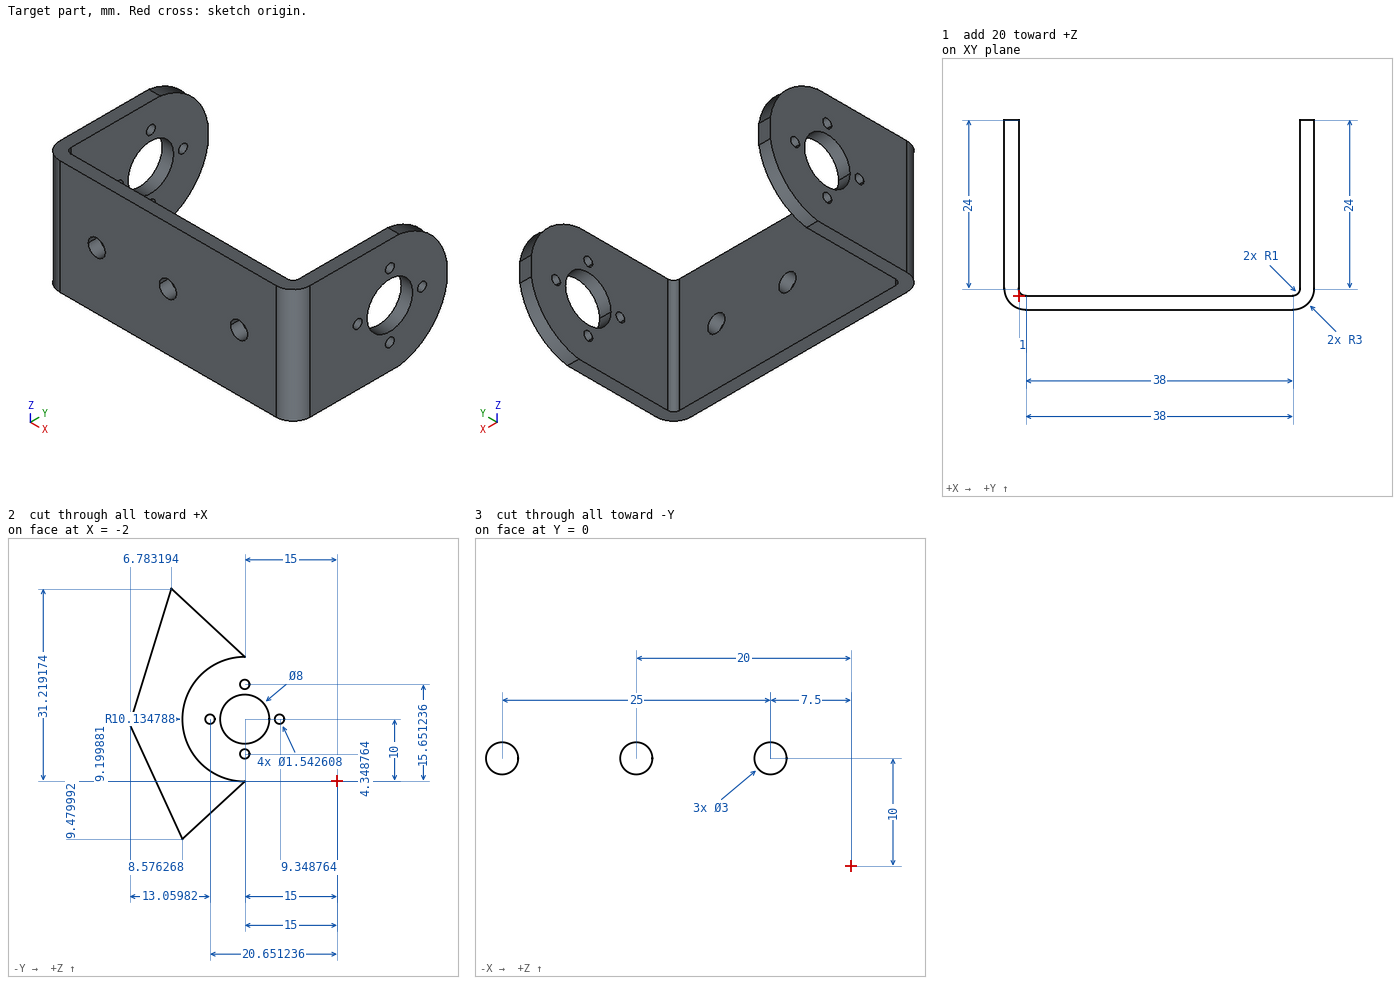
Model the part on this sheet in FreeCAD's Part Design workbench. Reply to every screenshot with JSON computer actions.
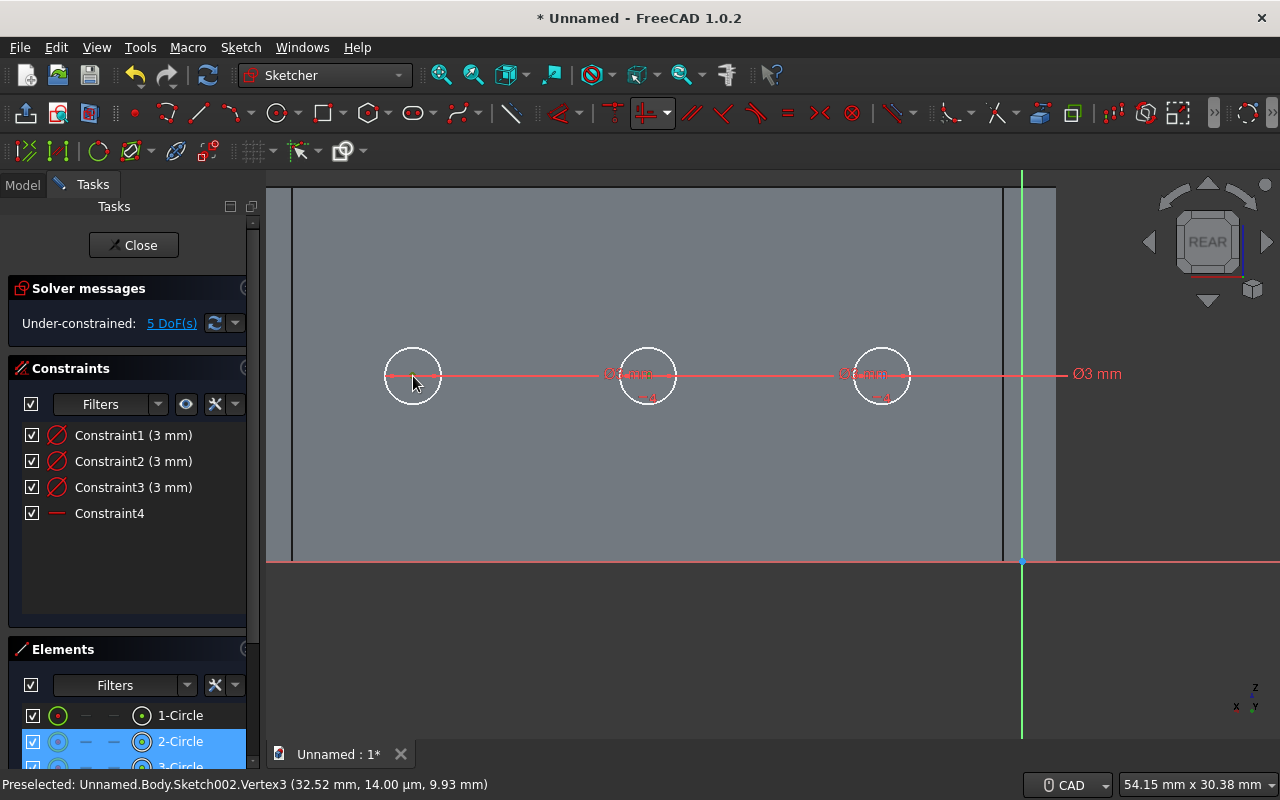
{"action": "left_click", "coordinate": [670, 114]}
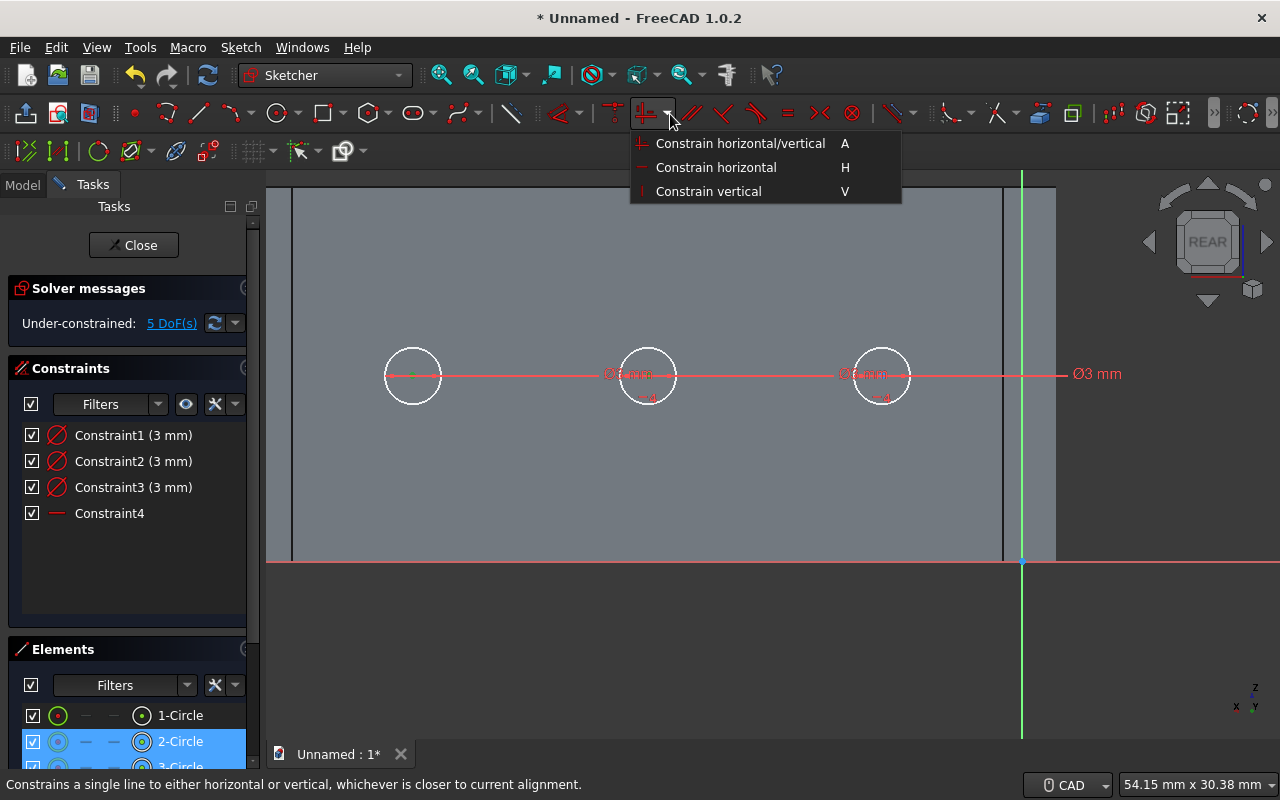
{"action": "left_click", "coordinate": [766, 167]}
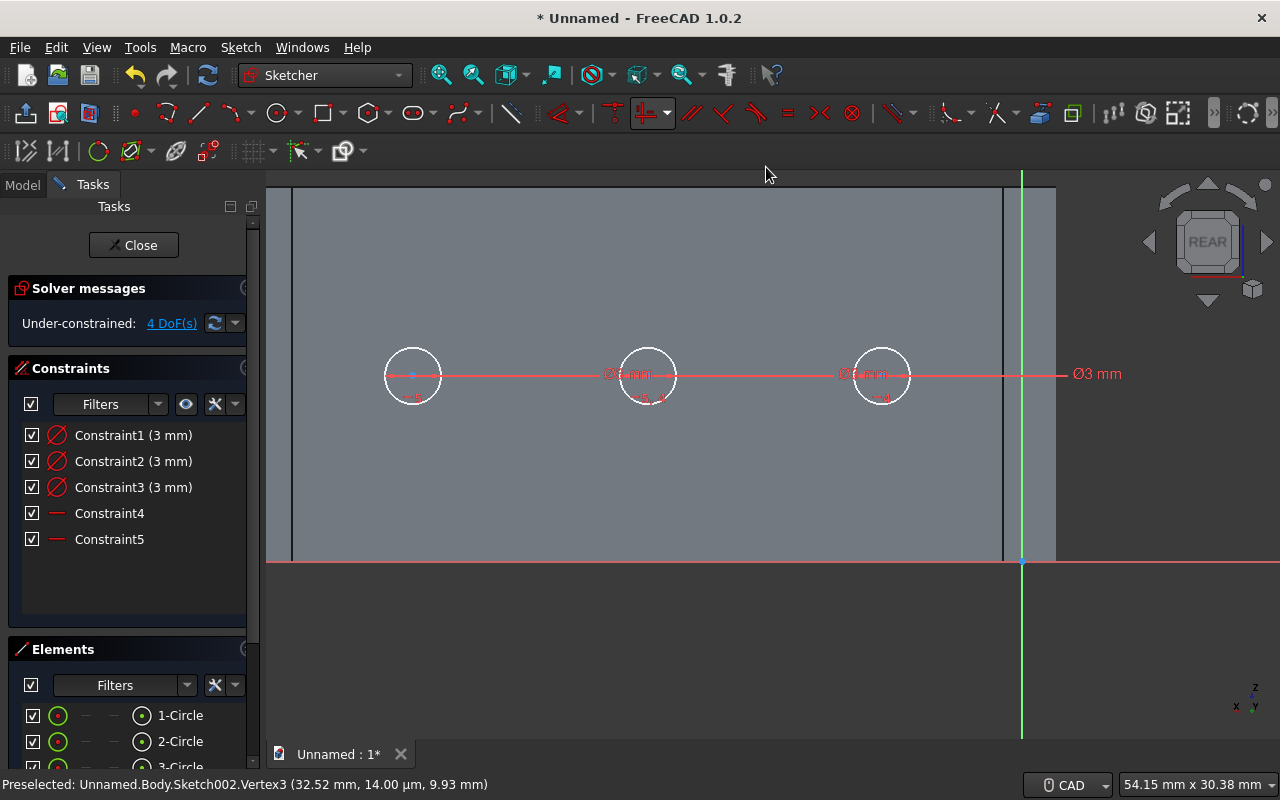
{"action": "left_click", "coordinate": [558, 114]}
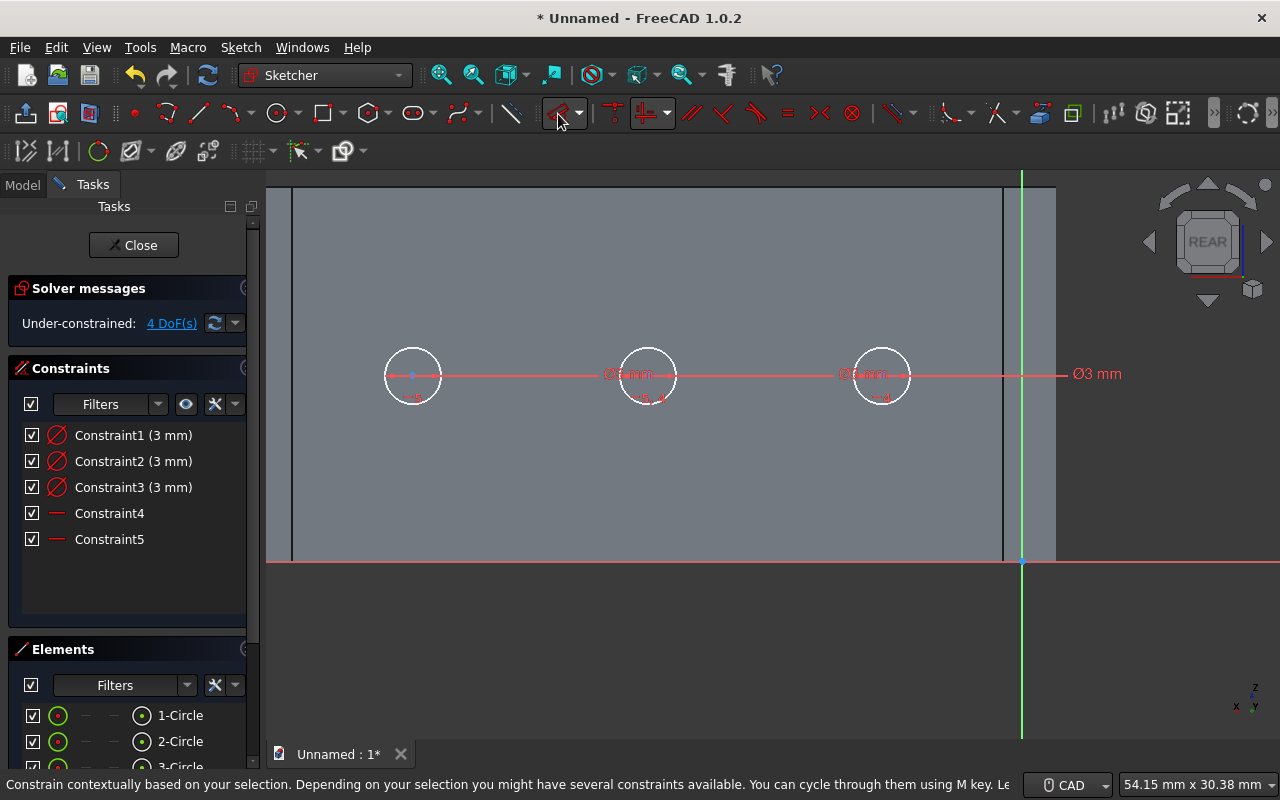
{"action": "left_click", "coordinate": [882, 376]}
{"action": "left_click", "coordinate": [1056, 469]}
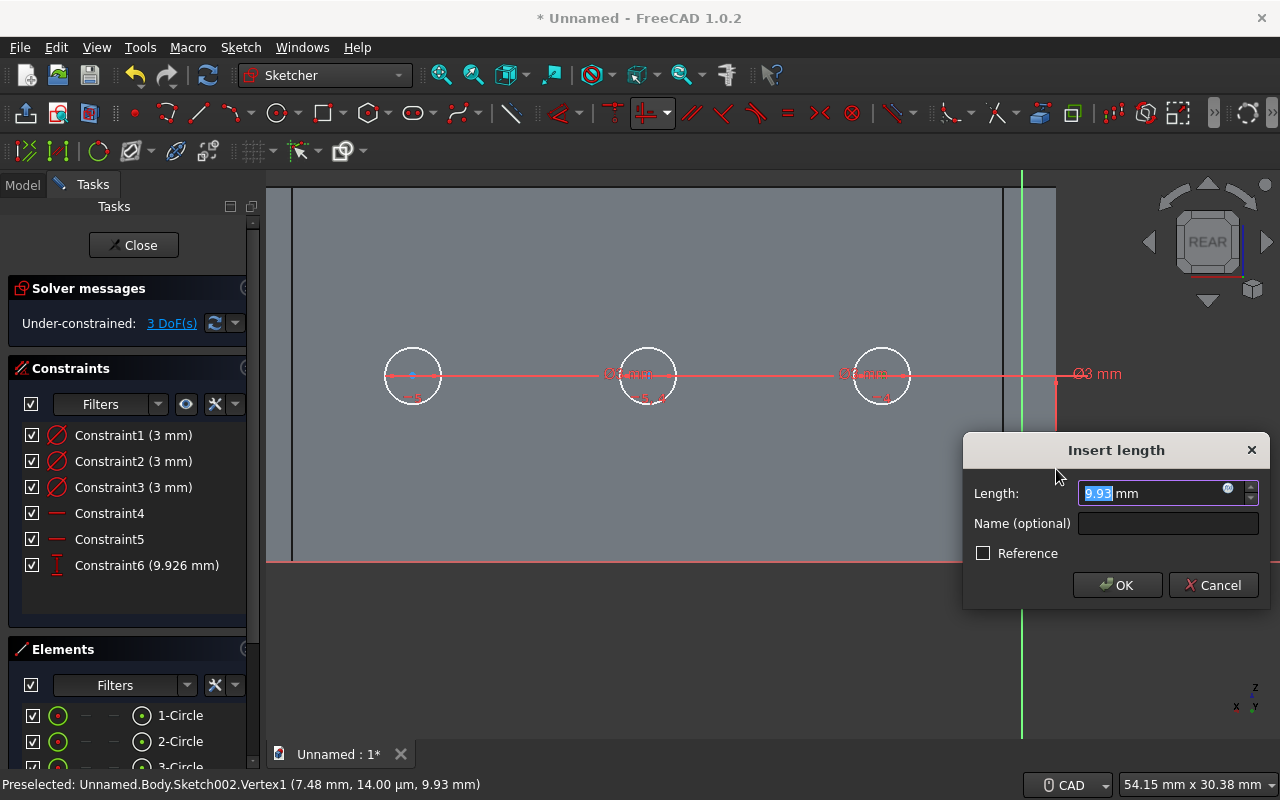
{"action": "type", "text": "10"}
{"action": "key", "text": "Return"}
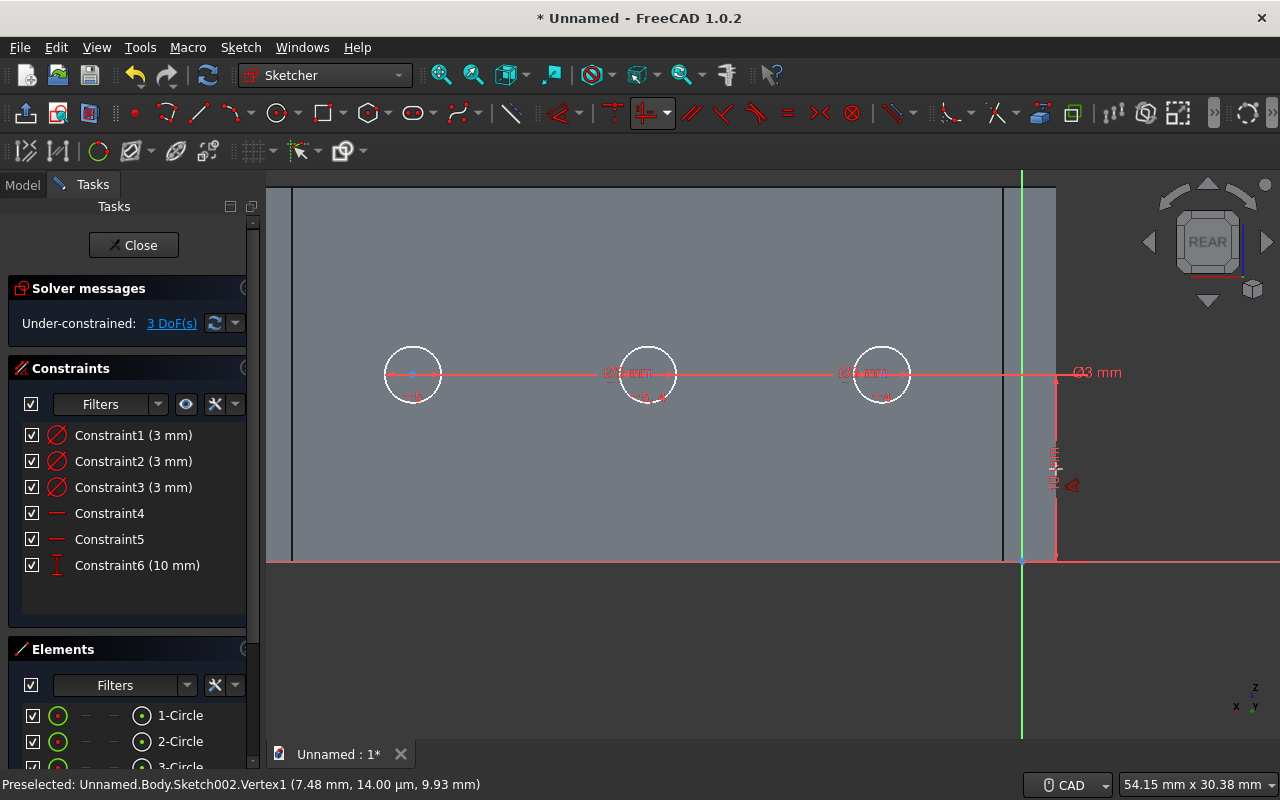
{"action": "left_click", "coordinate": [648, 375]}
{"action": "left_click", "coordinate": [835, 596]}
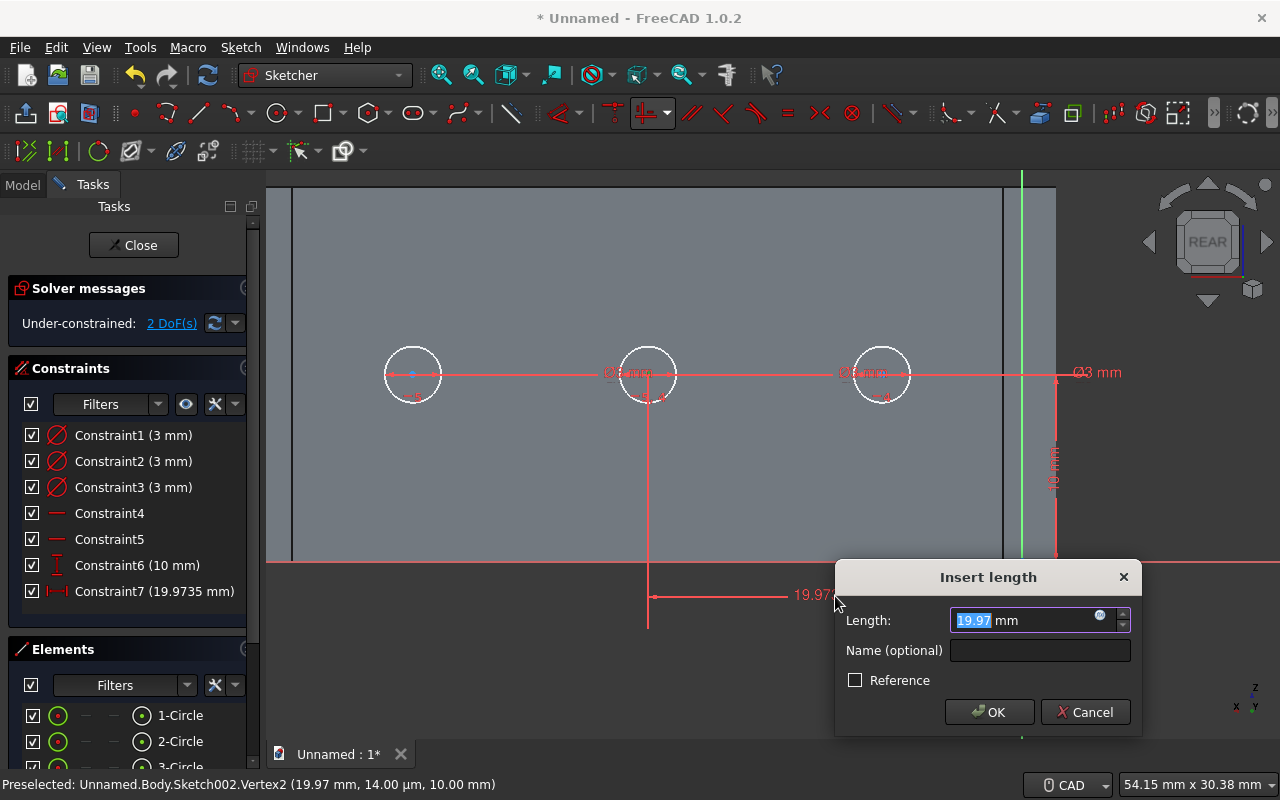
{"action": "type", "text": "20"}
{"action": "key", "text": "Return"}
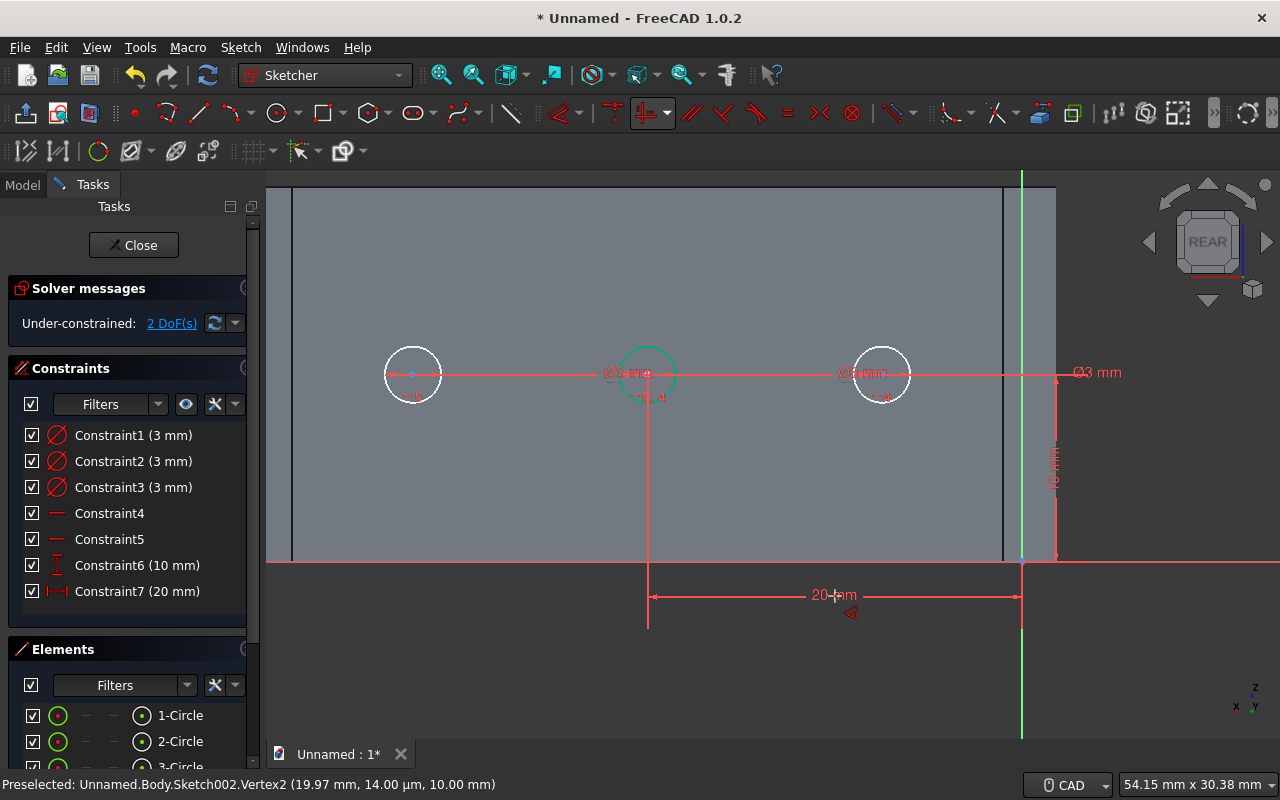
{"action": "left_click", "coordinate": [882, 375]}
{"action": "left_click", "coordinate": [952, 596]}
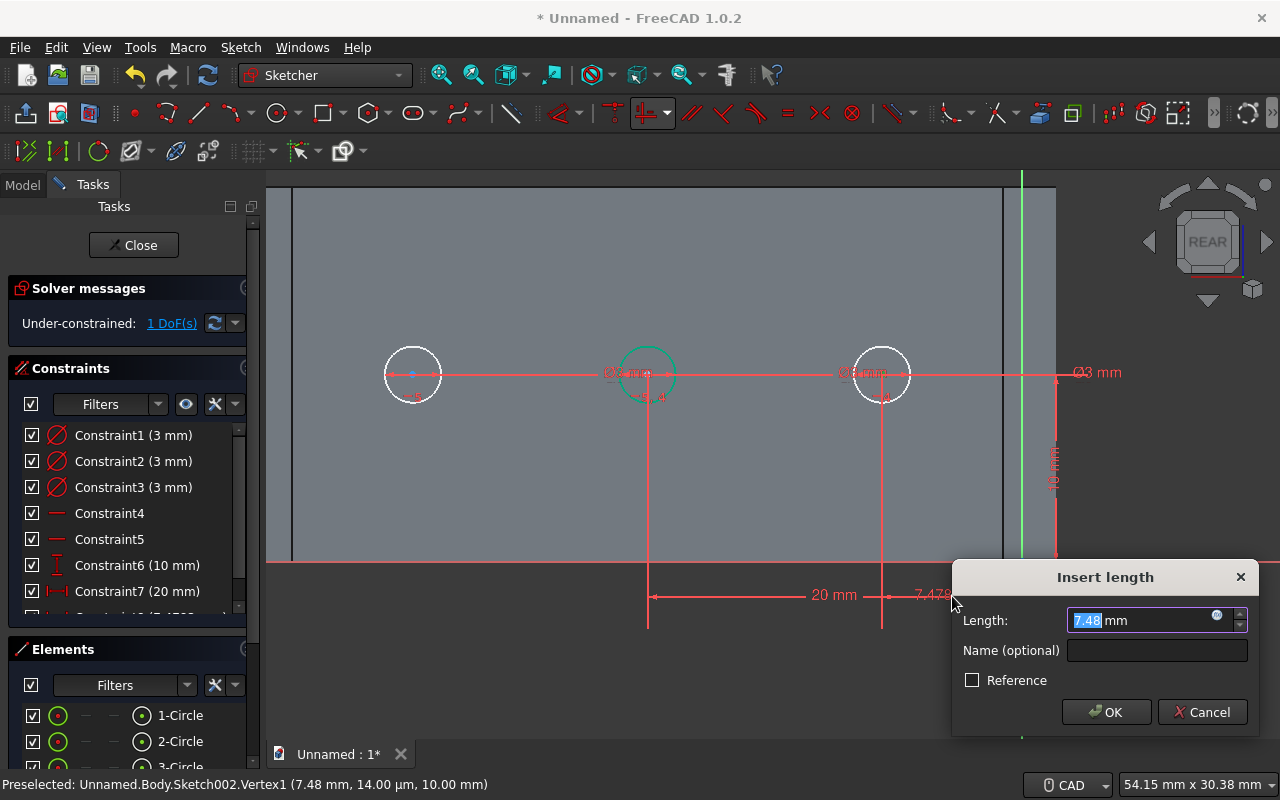
{"action": "type", "text": "7.5"}
{"action": "key", "text": "Return"}